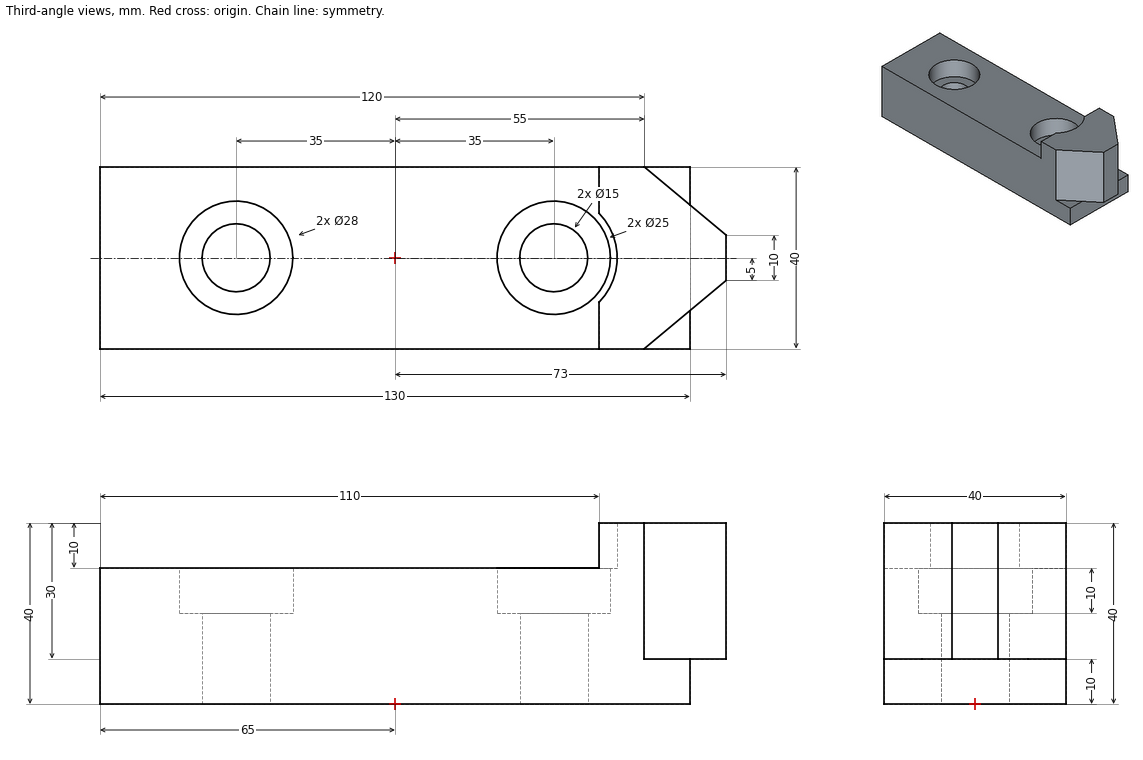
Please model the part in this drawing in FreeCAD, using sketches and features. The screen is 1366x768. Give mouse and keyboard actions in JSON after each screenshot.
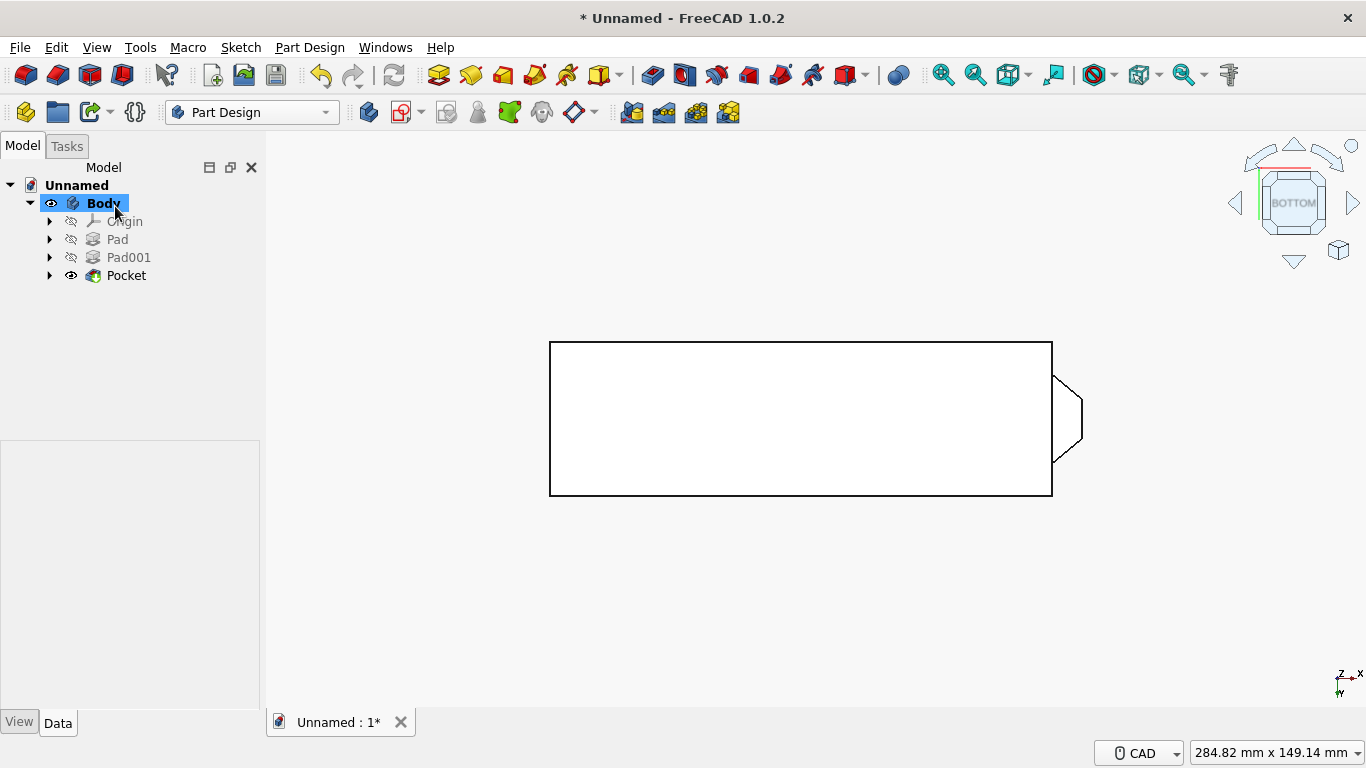
{"action": "left_click", "coordinate": [944, 418]}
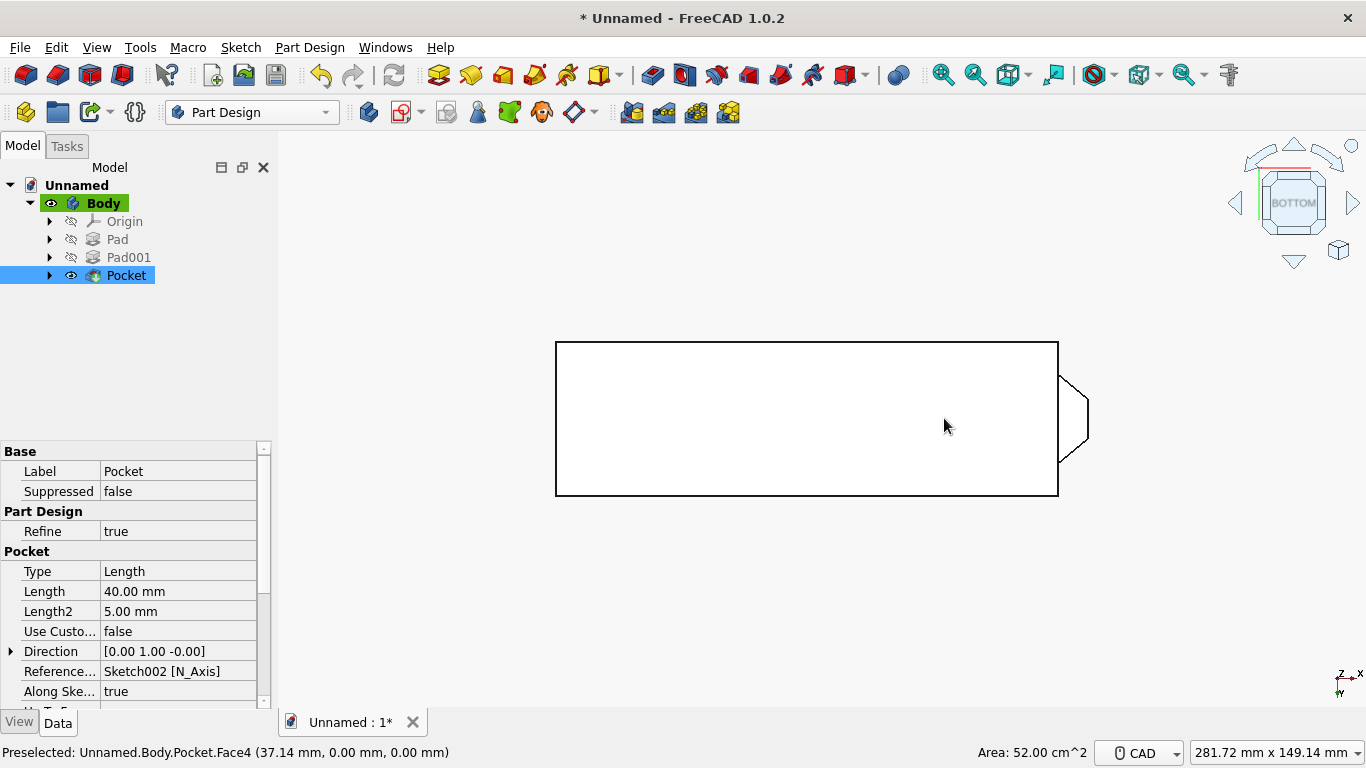
{"action": "left_click", "coordinate": [402, 112]}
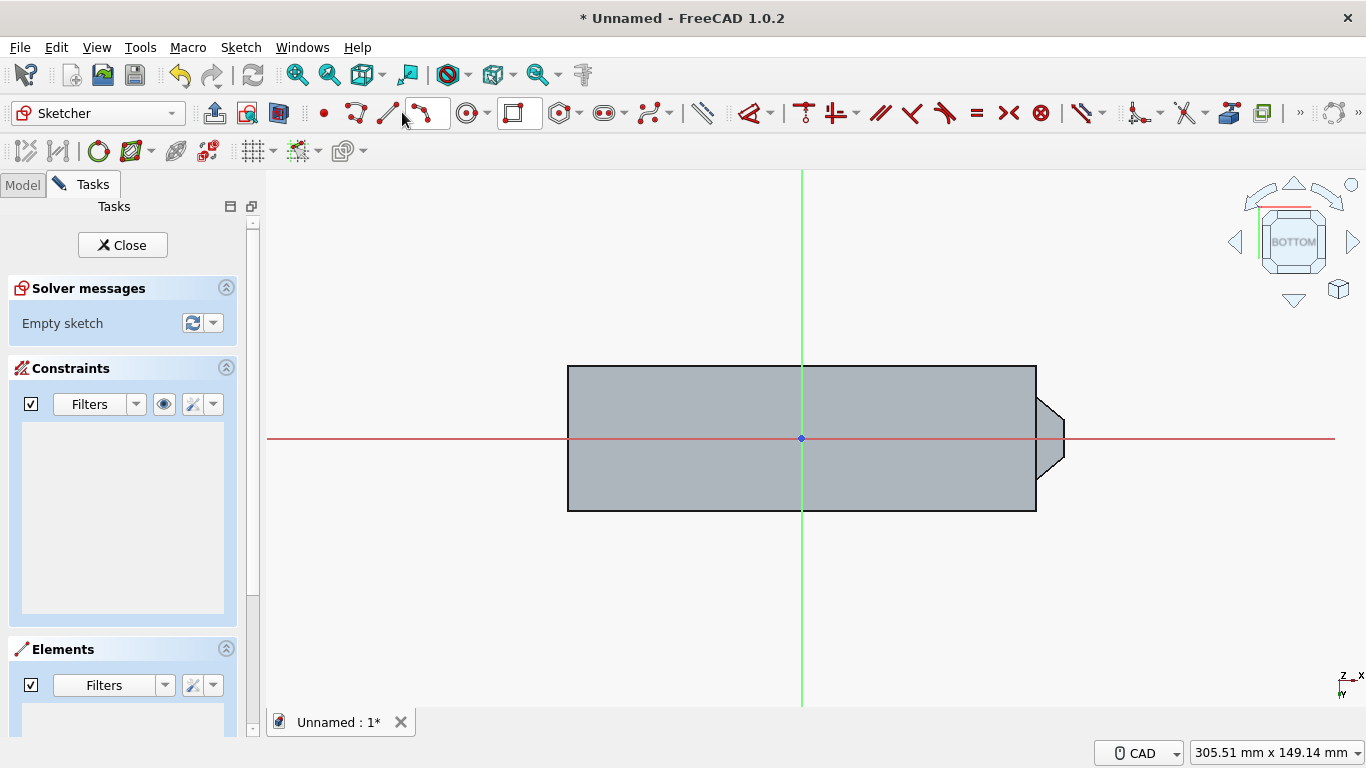
{"action": "scroll", "coordinate": [846, 438], "scroll_direction": "up", "scroll_amount": 4}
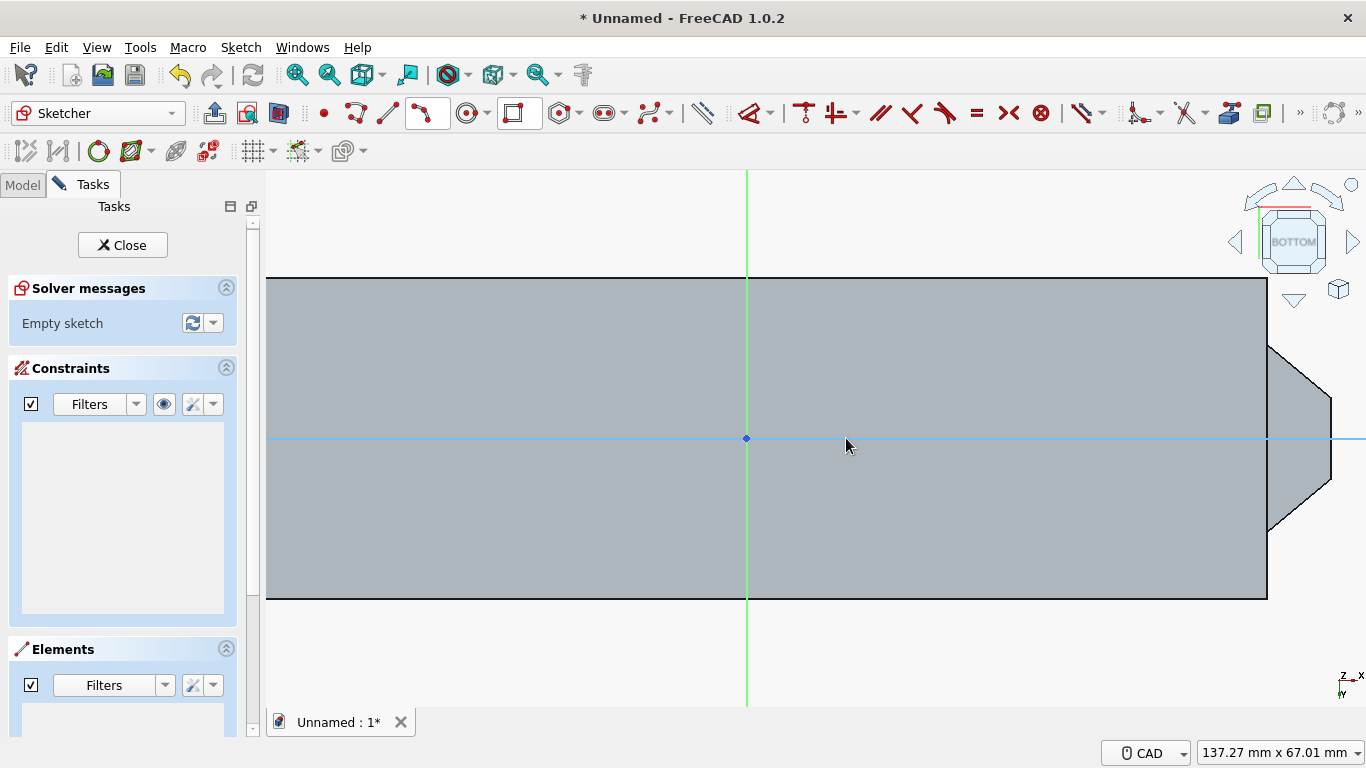
{"action": "left_click", "coordinate": [468, 114]}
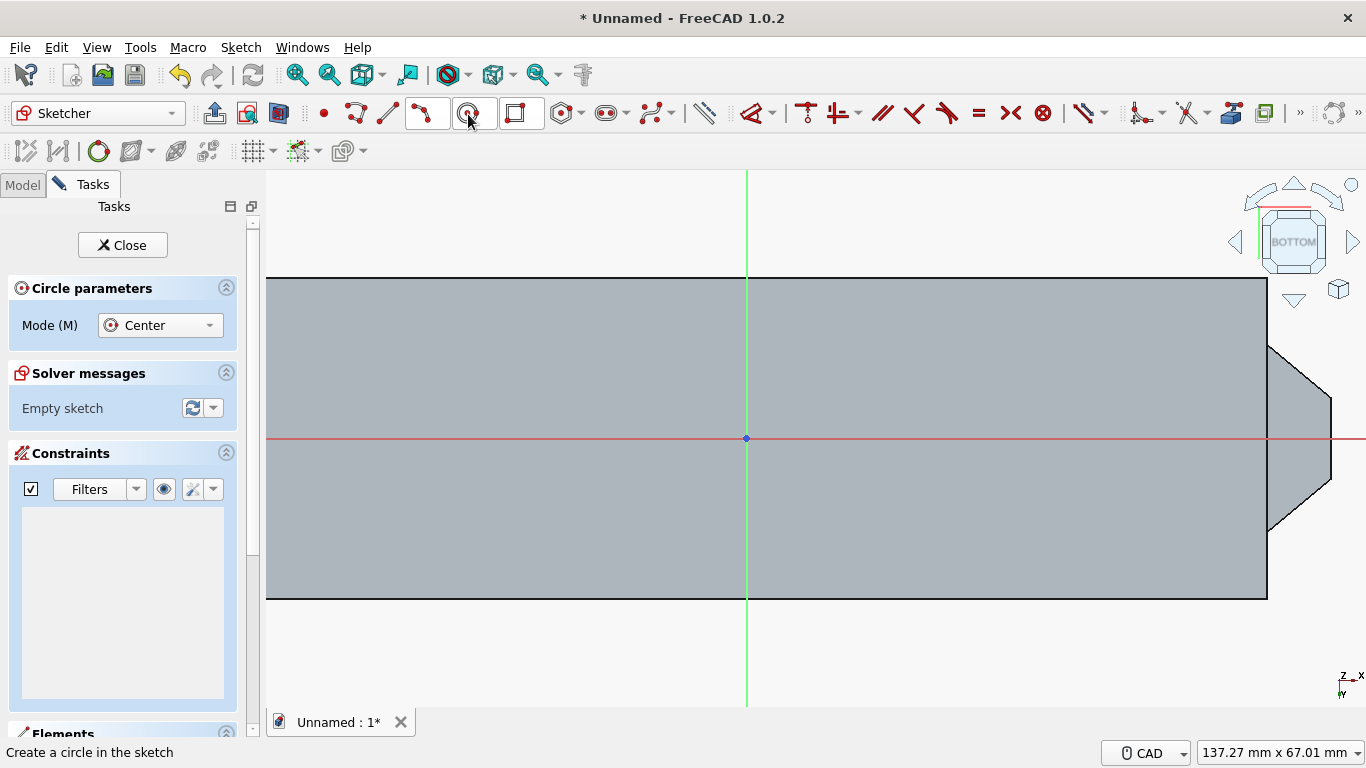
{"action": "left_click", "coordinate": [1027, 438]}
{"action": "left_click", "coordinate": [1069, 396]}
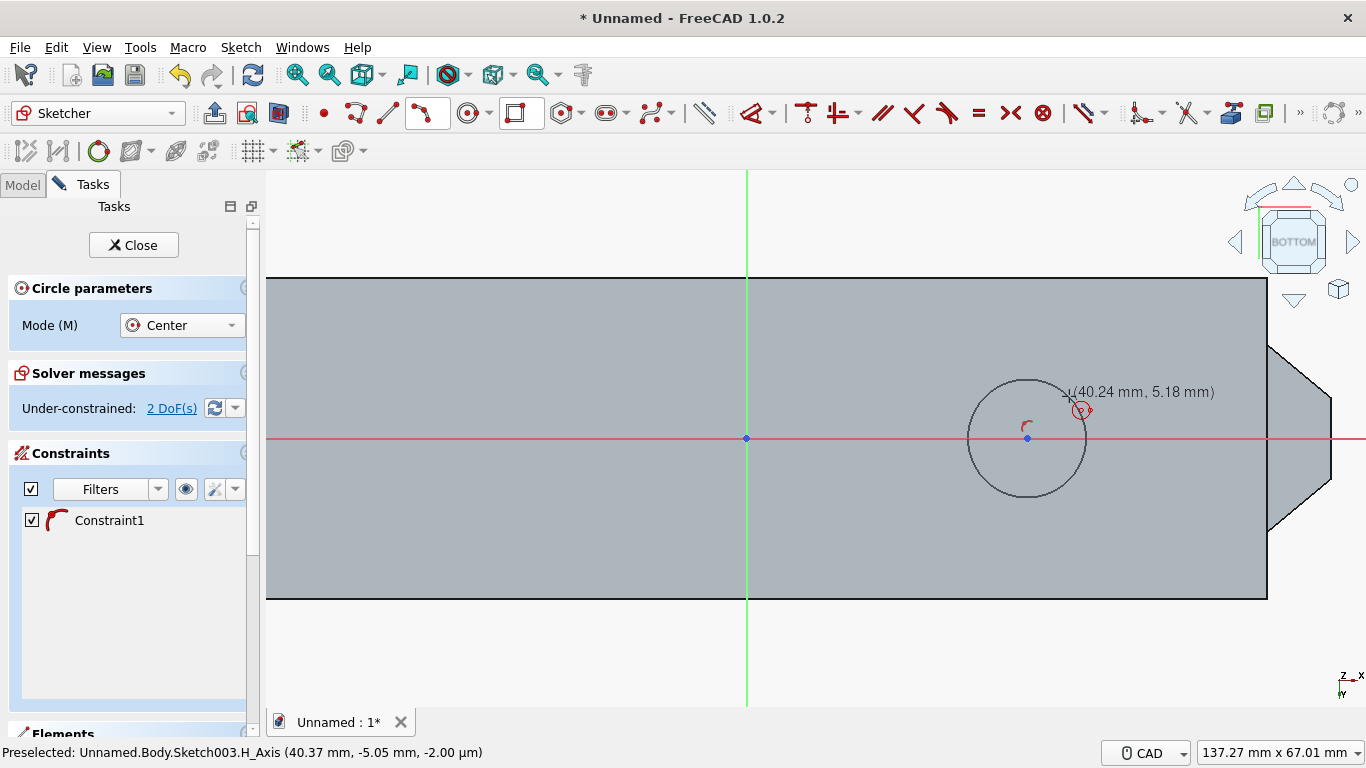
{"action": "left_click", "coordinate": [466, 438]}
{"action": "left_click", "coordinate": [509, 396]}
{"action": "key", "text": "Escape"}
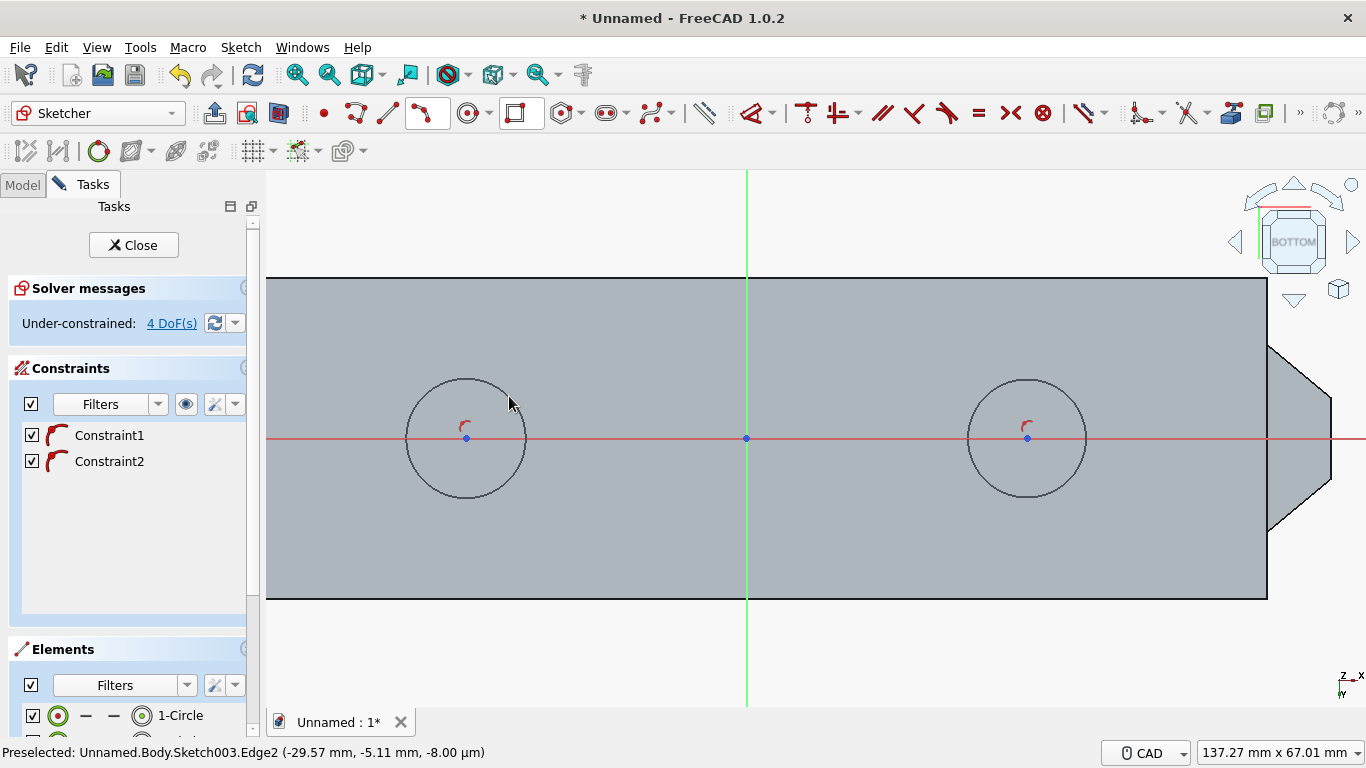
{"action": "left_click", "coordinate": [1069, 397]}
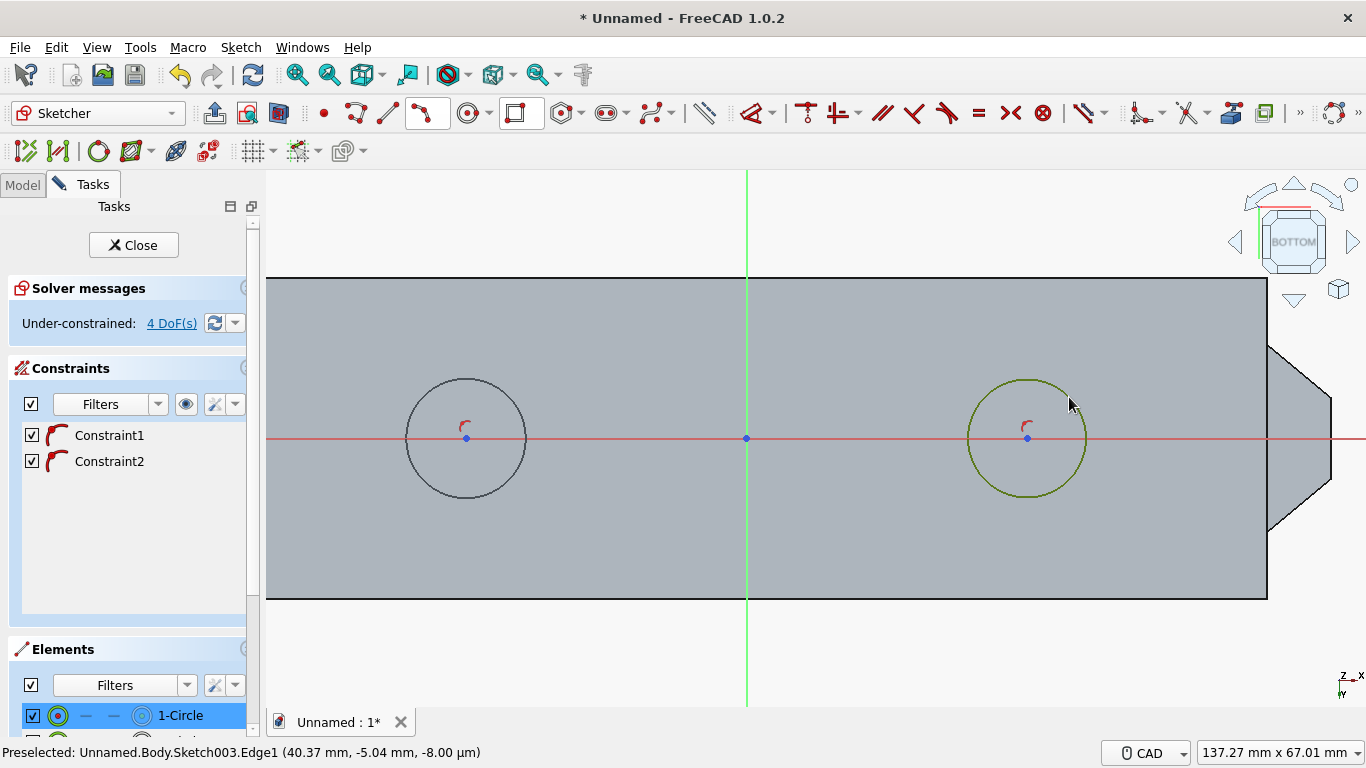
{"action": "left_click", "coordinate": [508, 396]}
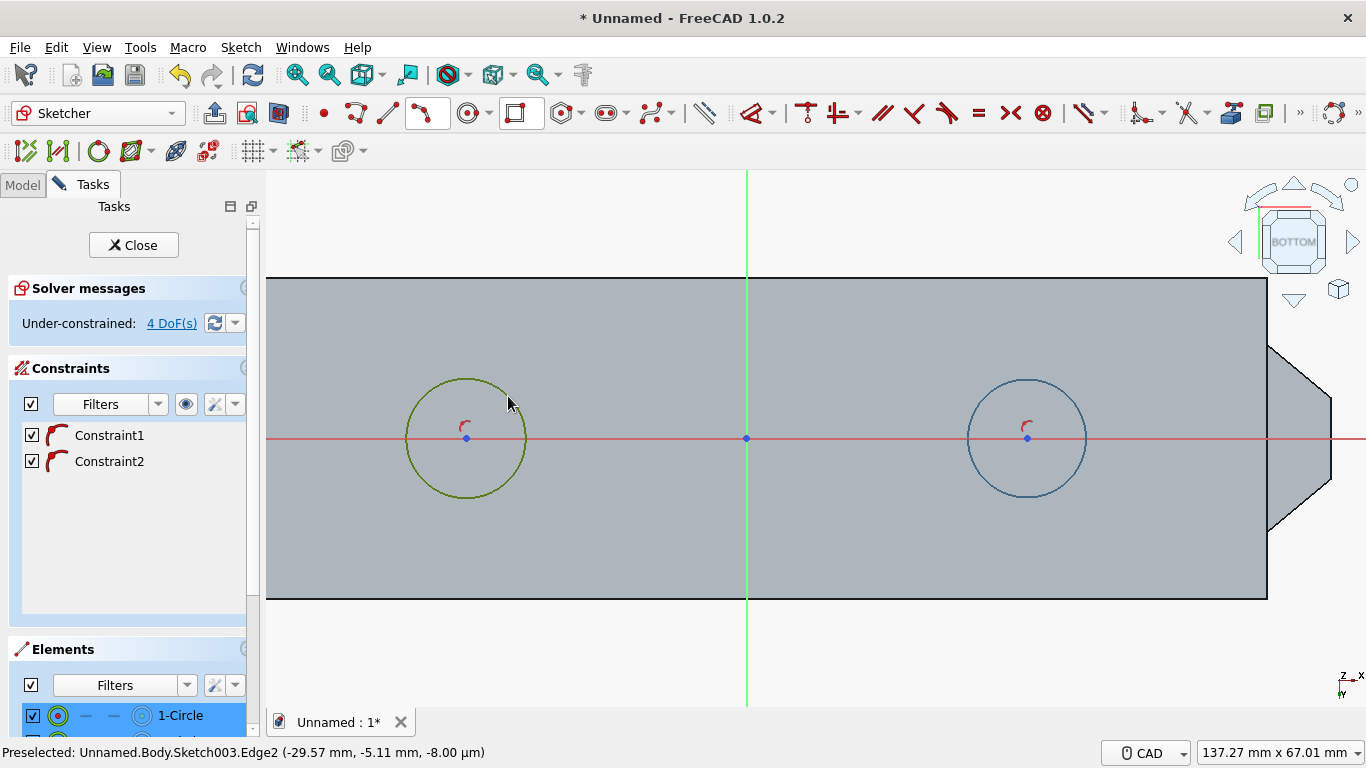
{"action": "left_click", "coordinate": [980, 114]}